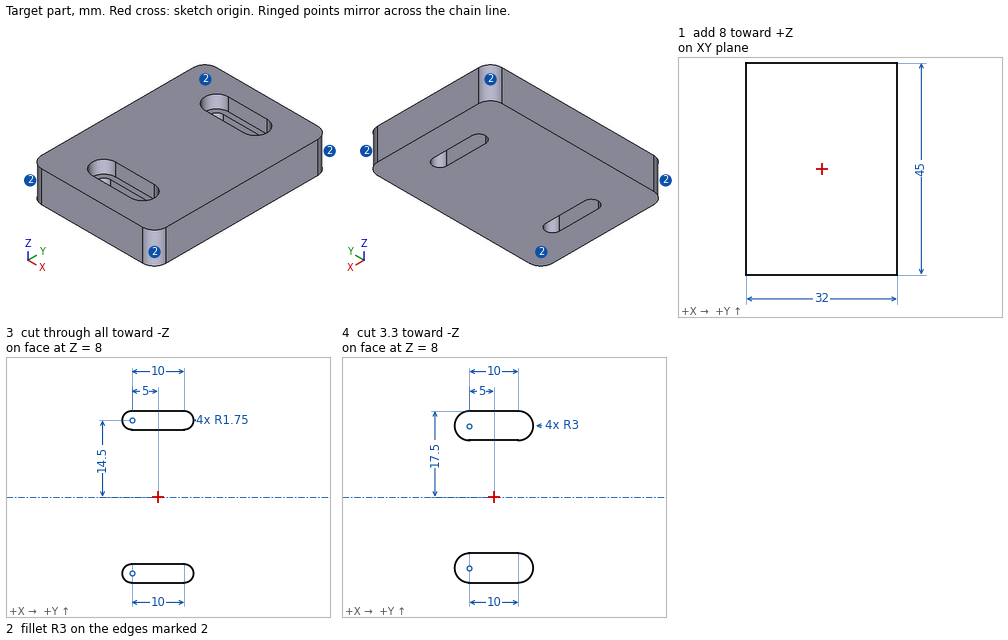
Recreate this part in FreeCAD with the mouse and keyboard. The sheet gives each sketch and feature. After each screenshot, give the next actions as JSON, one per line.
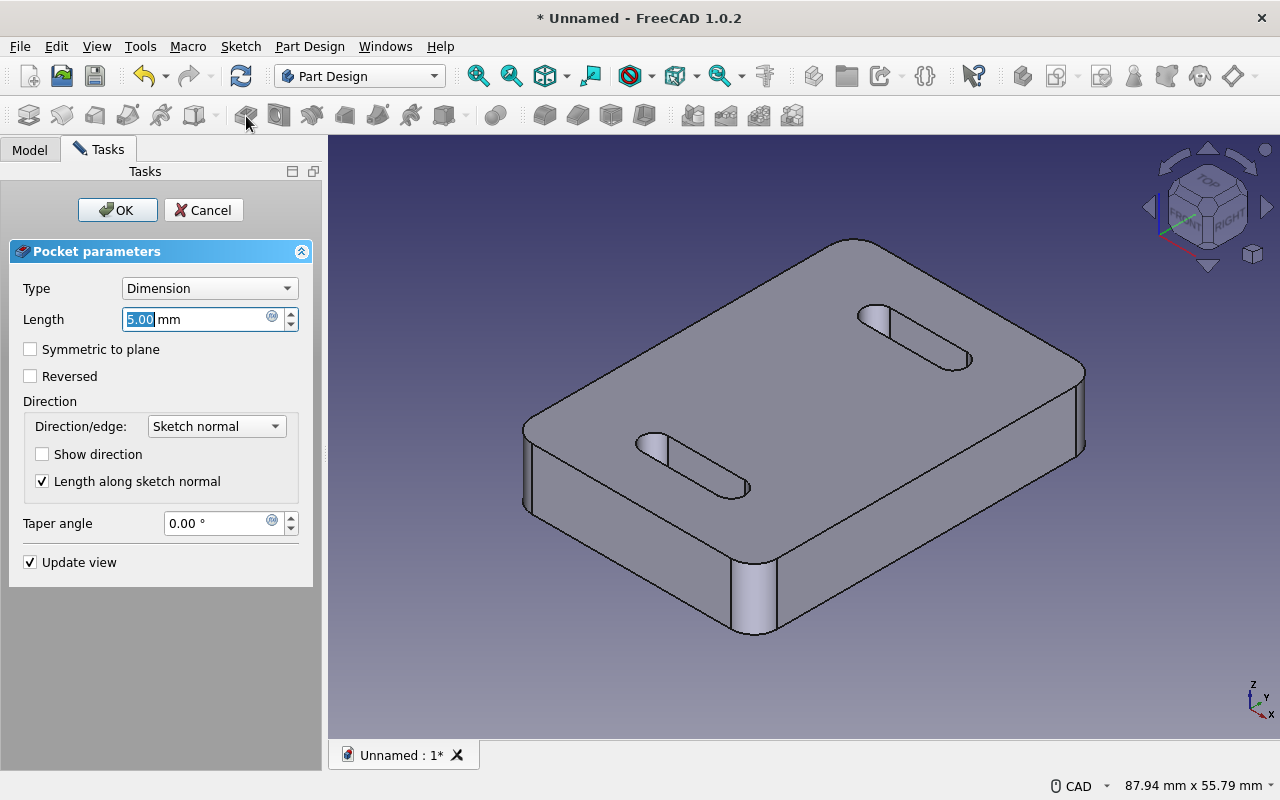
{"action": "left_click", "coordinate": [210, 288]}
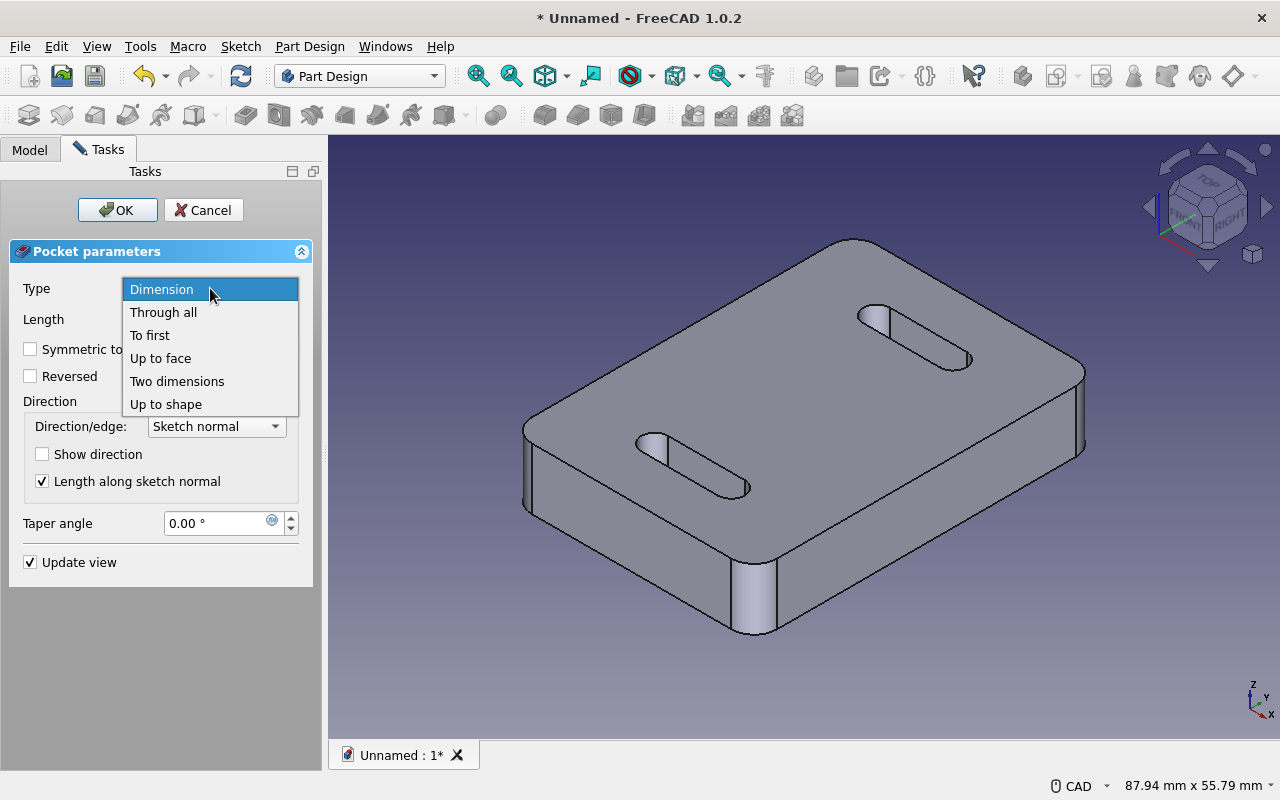
{"action": "left_click", "coordinate": [208, 312]}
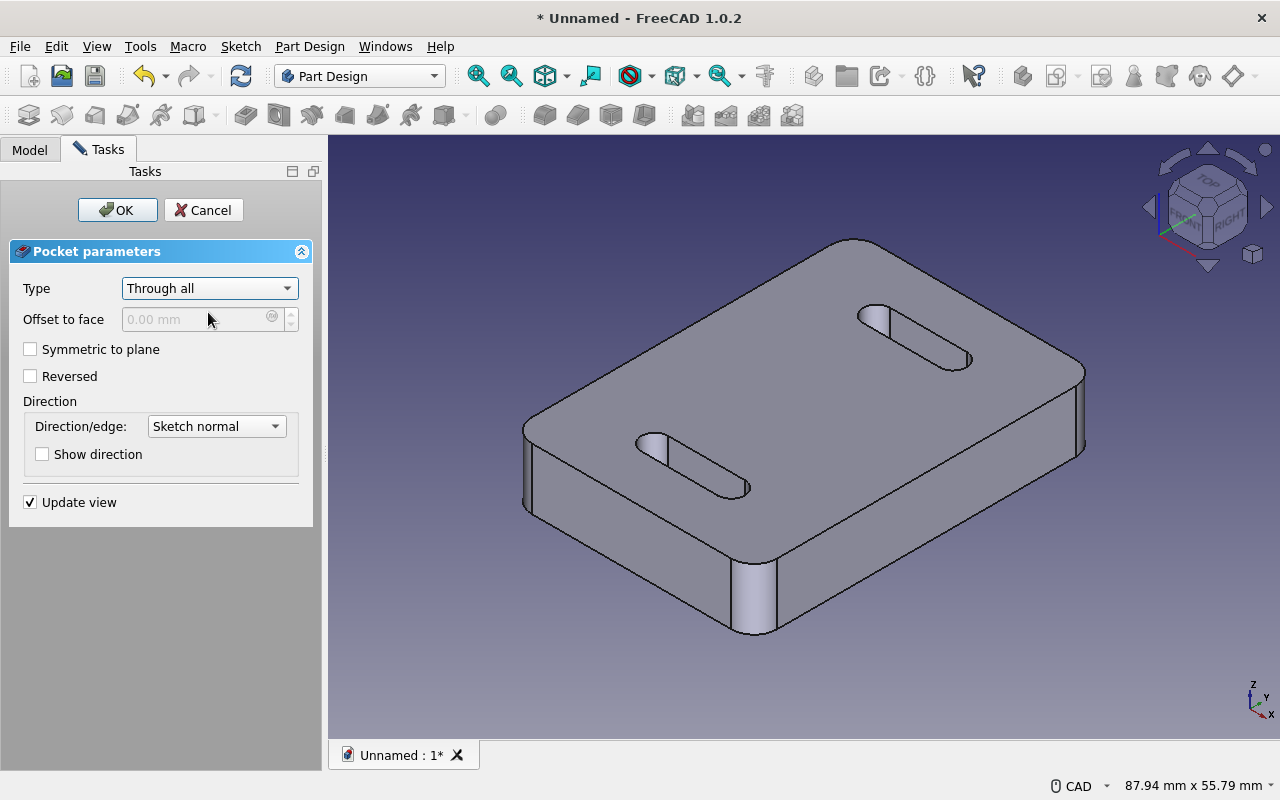
{"action": "left_click", "coordinate": [118, 210]}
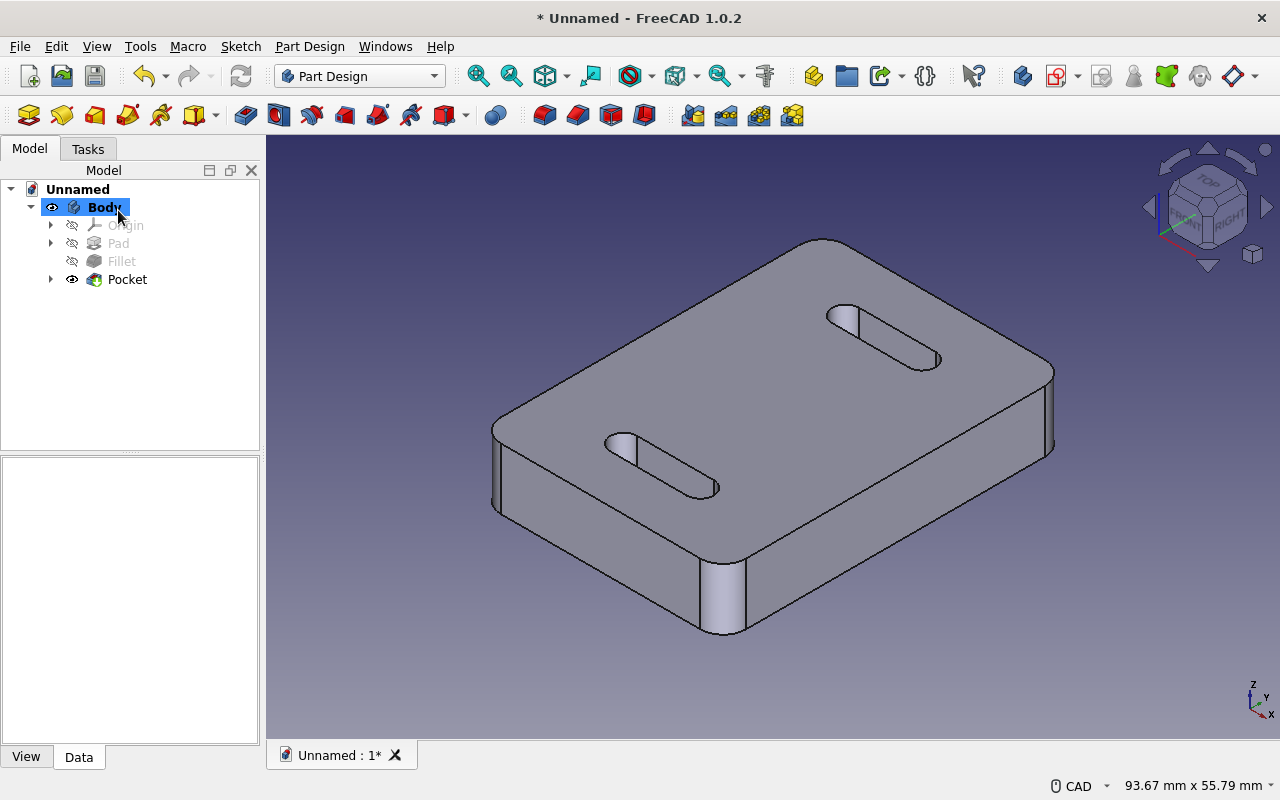
{"action": "left_click", "coordinate": [773, 401]}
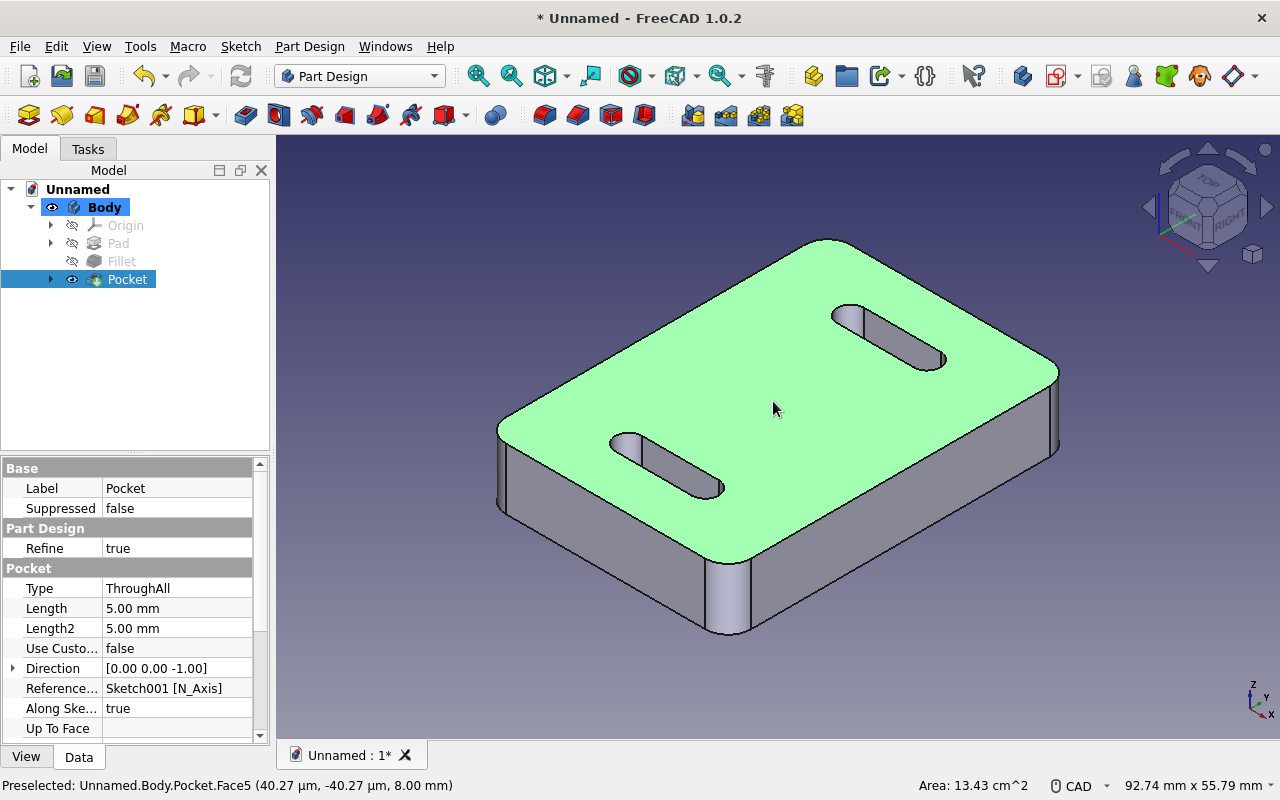
{"action": "left_click", "coordinate": [1056, 76]}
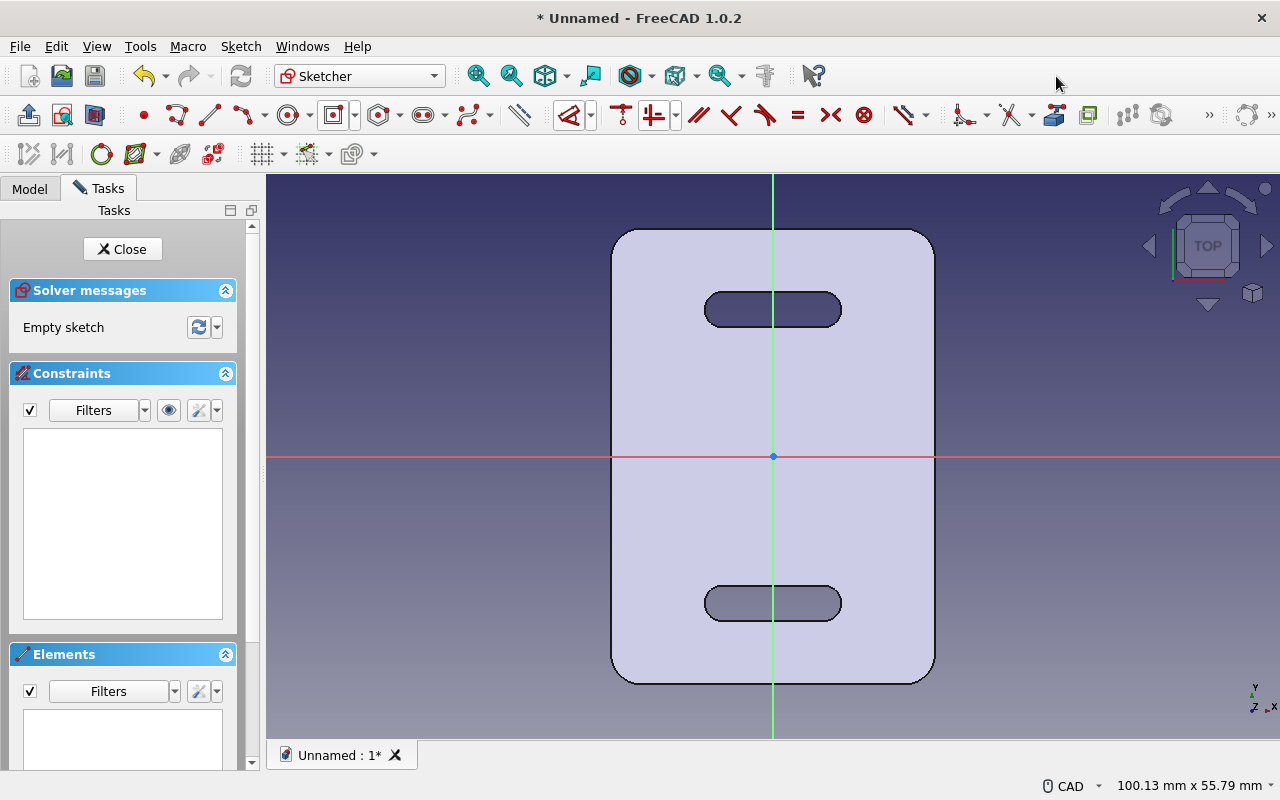
{"action": "left_click", "coordinate": [422, 116]}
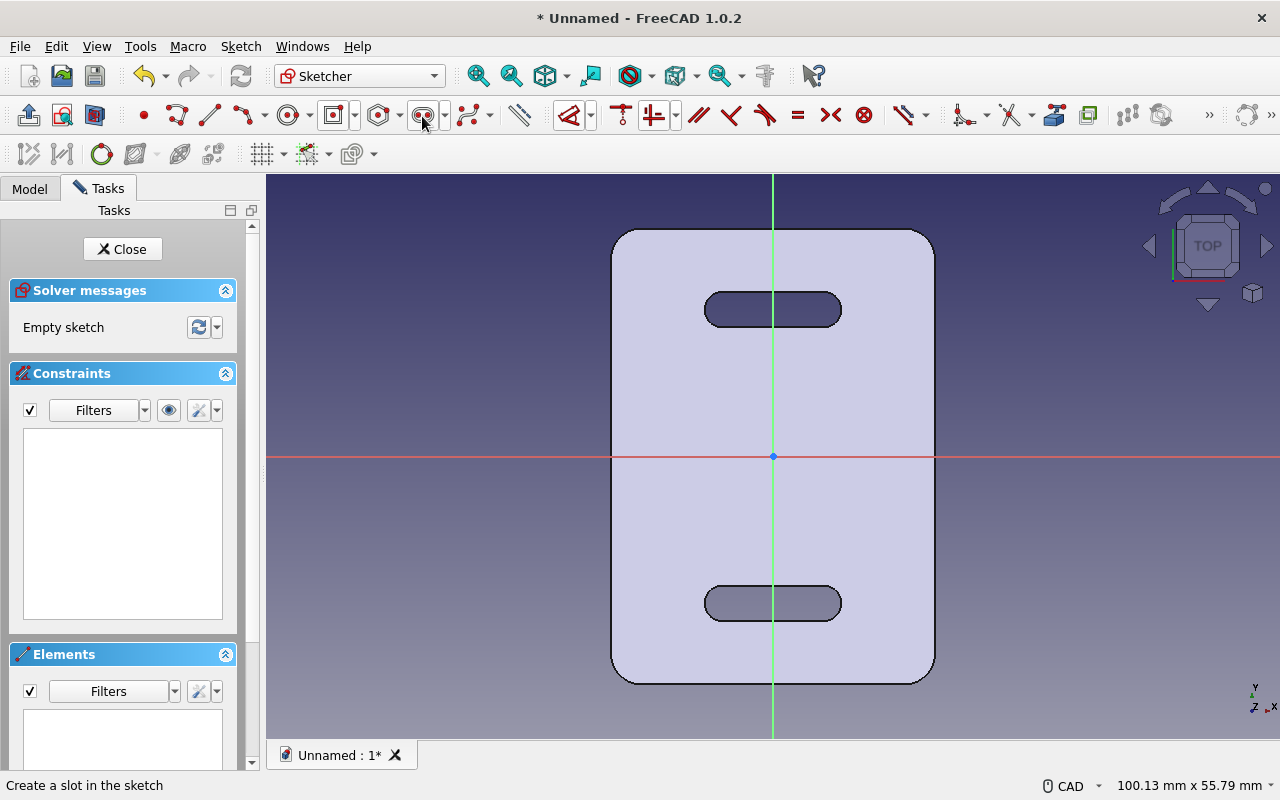
{"action": "left_click", "coordinate": [722, 310]}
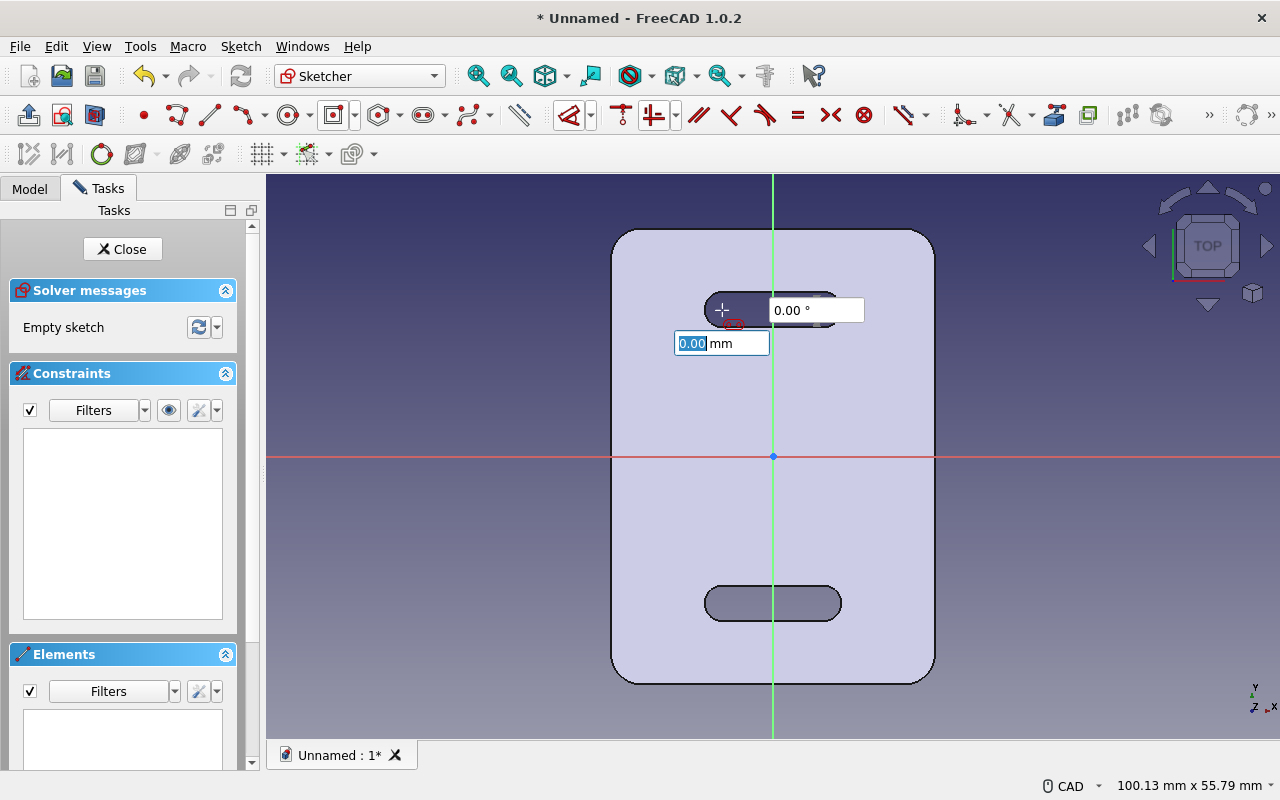
{"action": "left_click", "coordinate": [824, 310]}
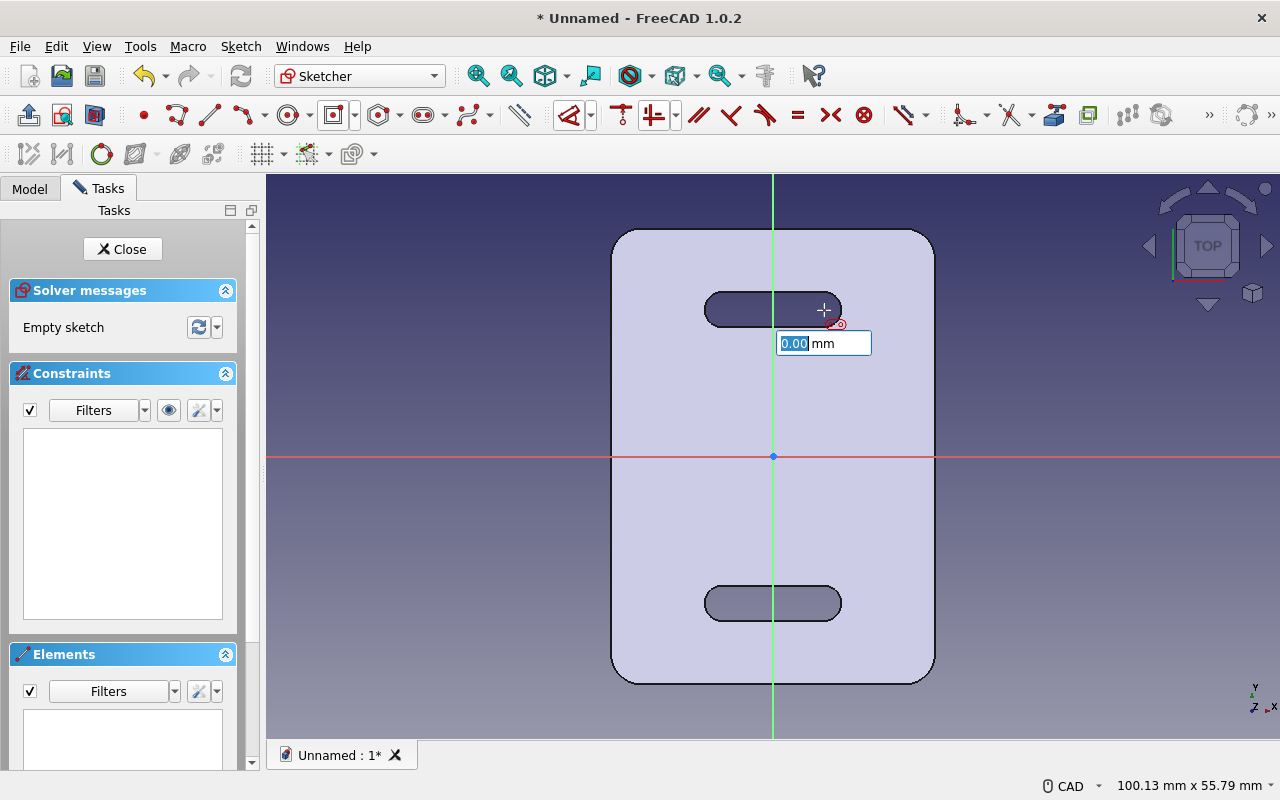
{"action": "left_click", "coordinate": [788, 279]}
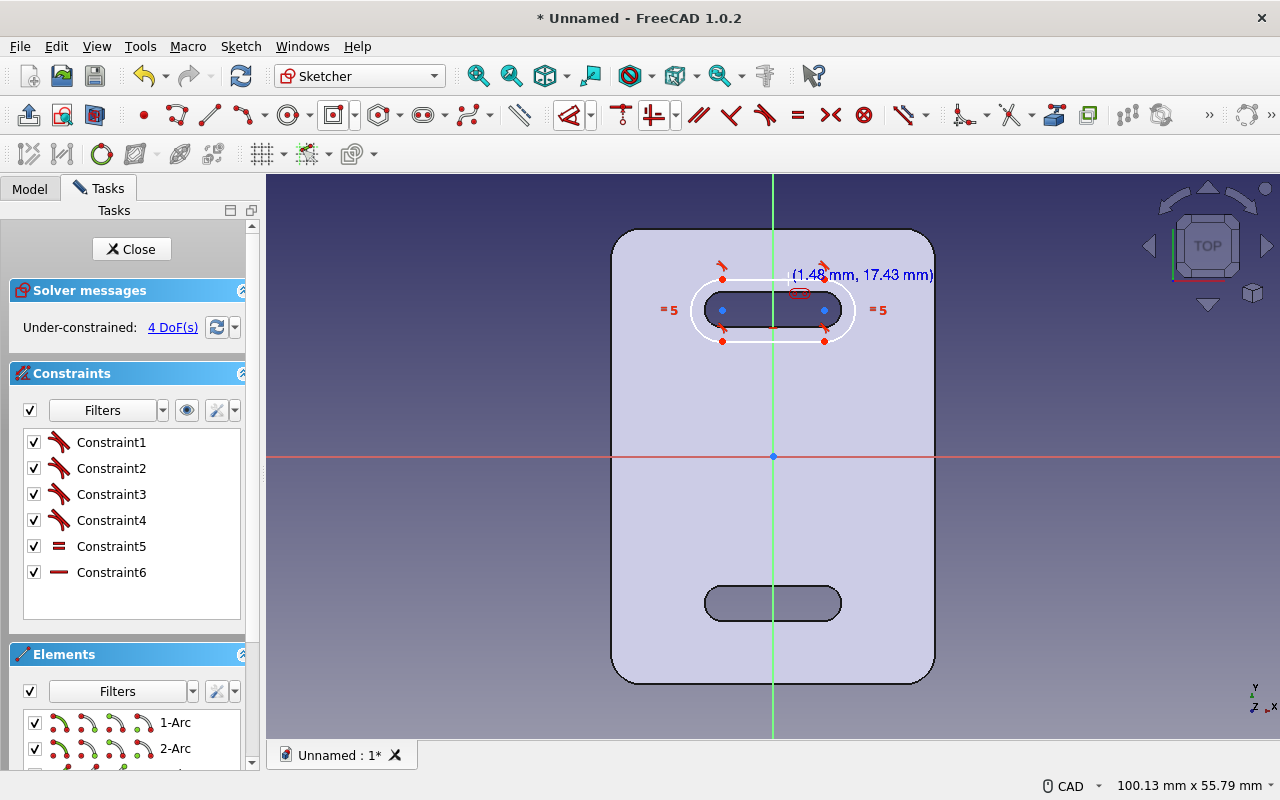
{"action": "left_click", "coordinate": [722, 603]}